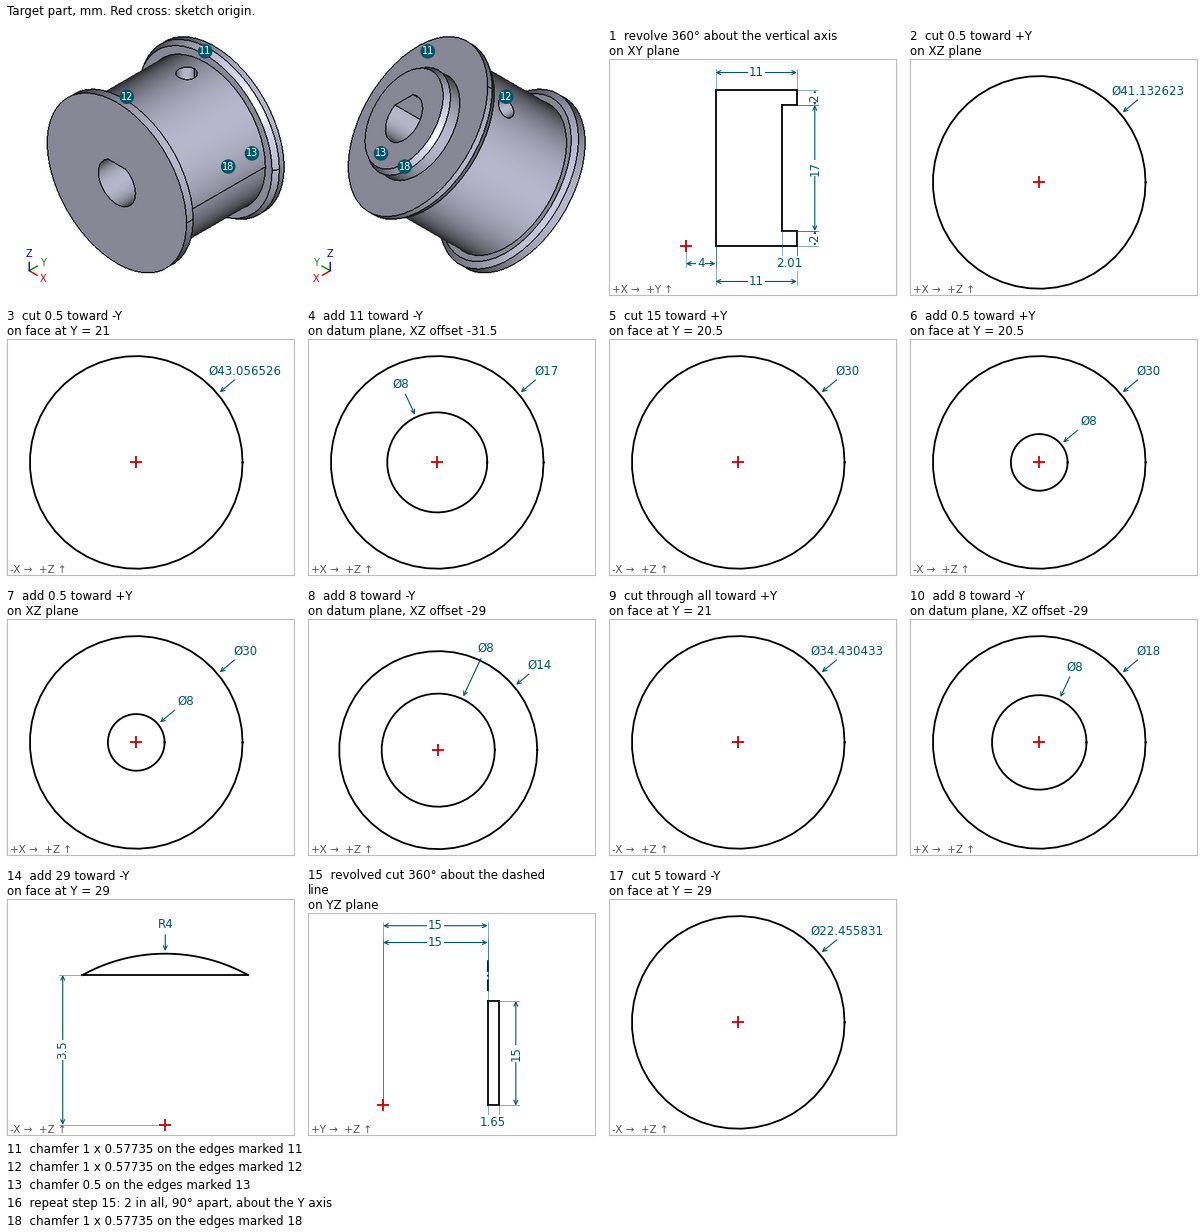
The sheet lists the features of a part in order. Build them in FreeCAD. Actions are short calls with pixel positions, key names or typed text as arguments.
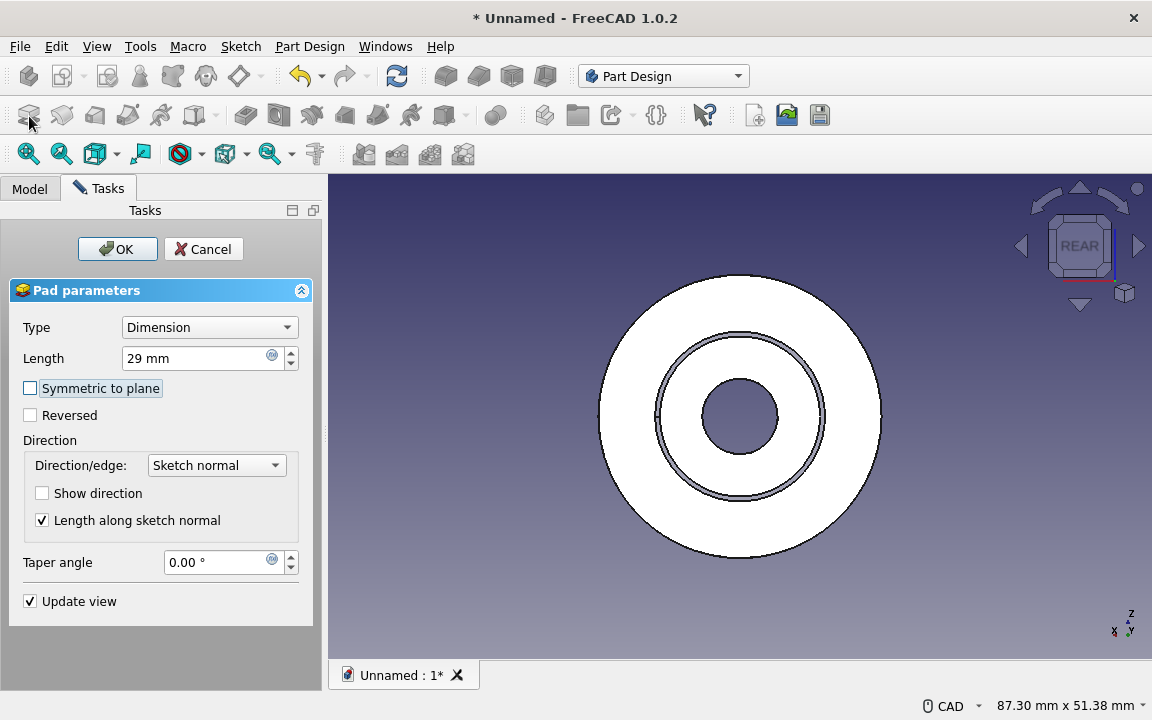
click(31, 415)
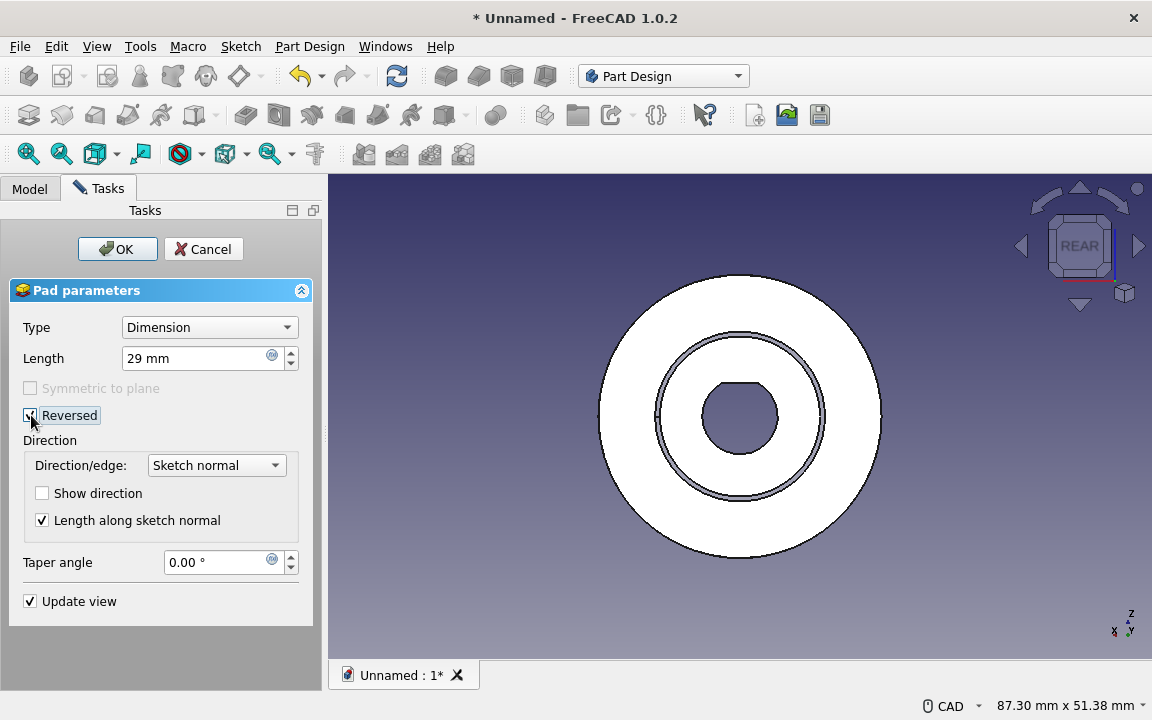
click(118, 249)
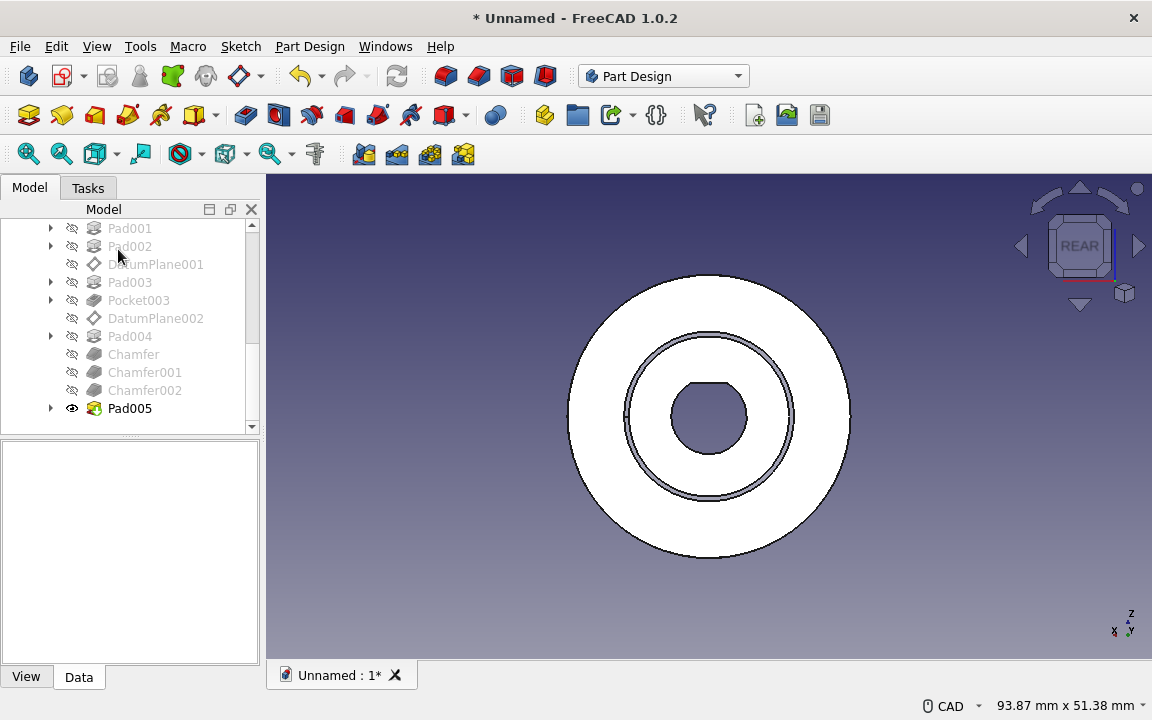
click(62, 76)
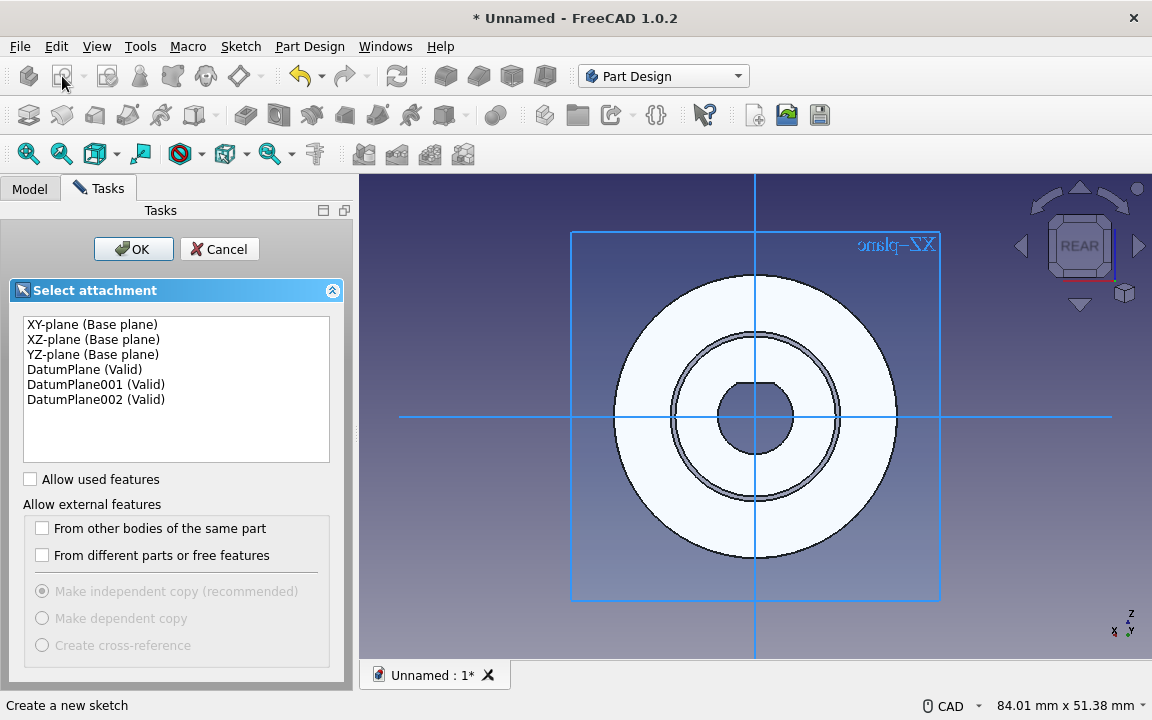
click(84, 354)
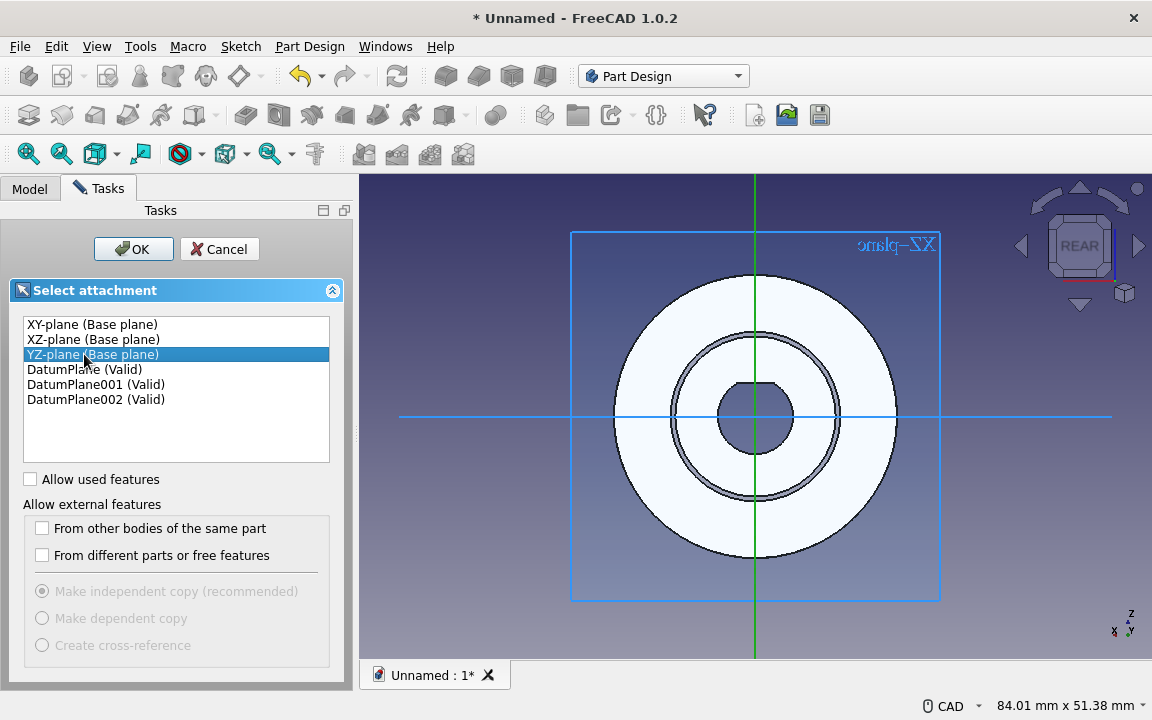
click(134, 249)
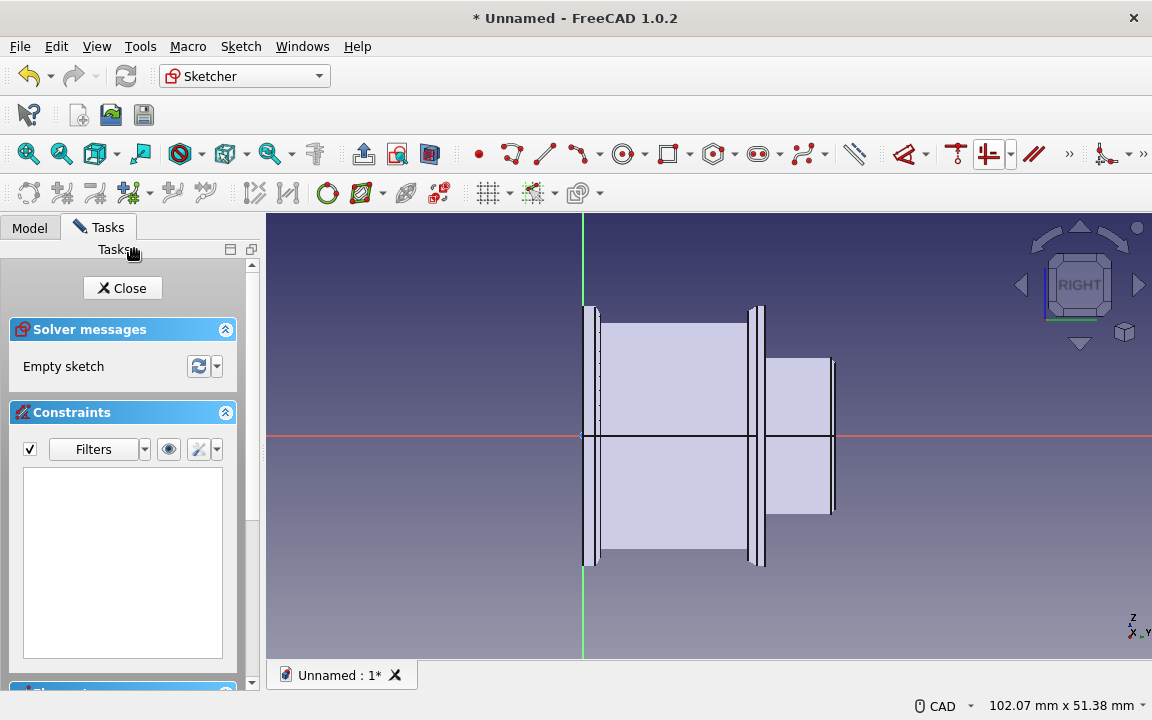
click(430, 154)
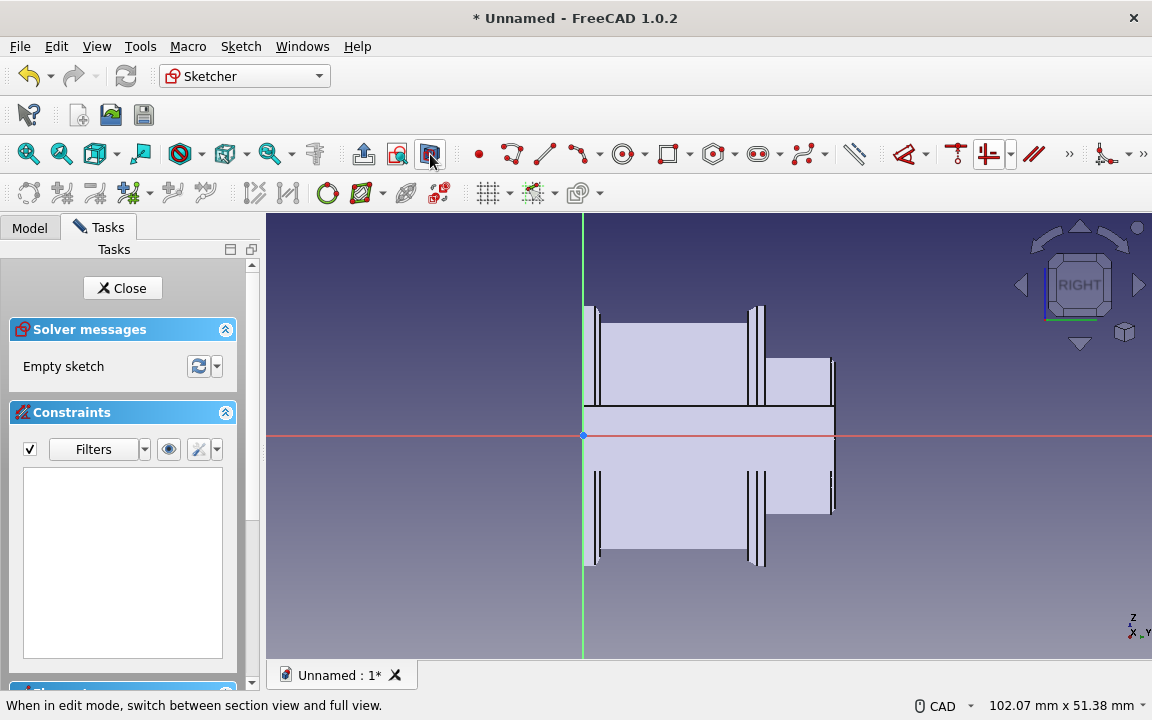
scroll(573, 631, down, 1)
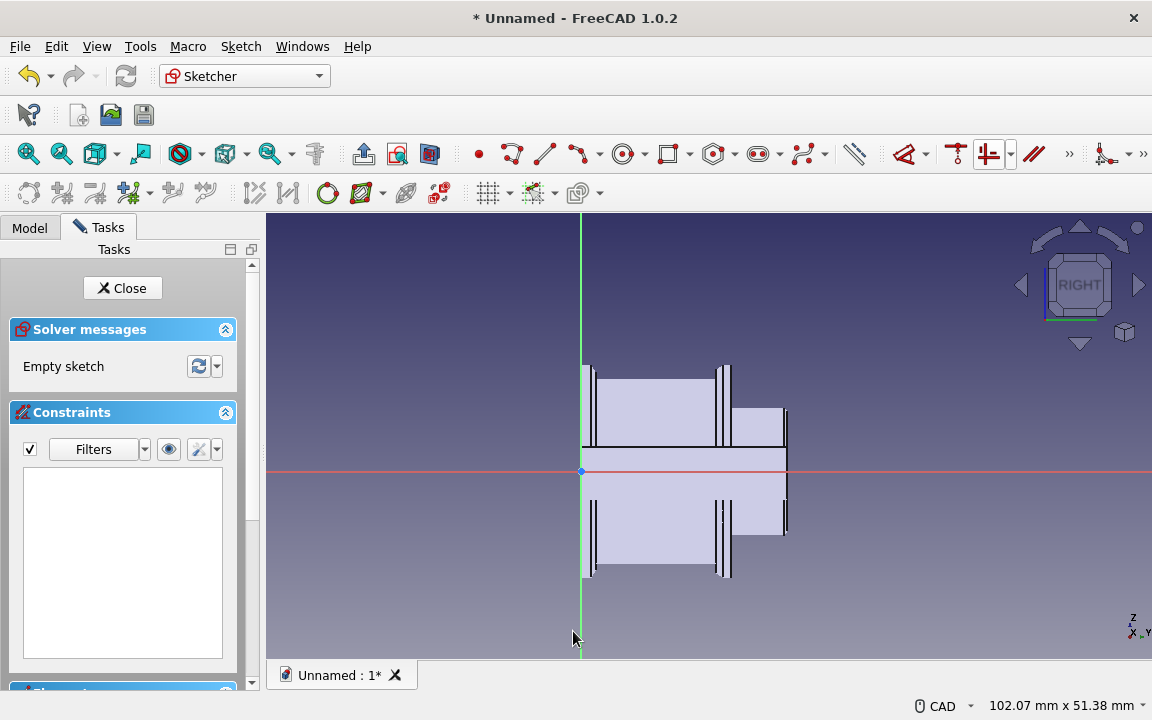
scroll(641, 349, up, 3)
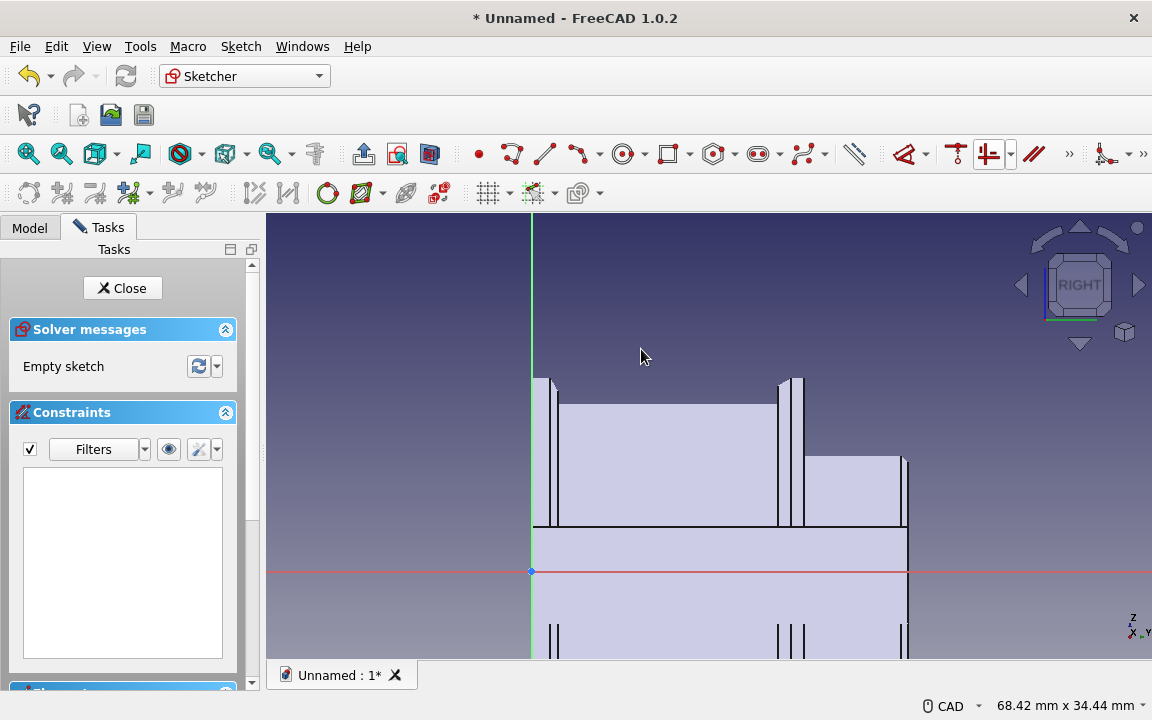
click(668, 154)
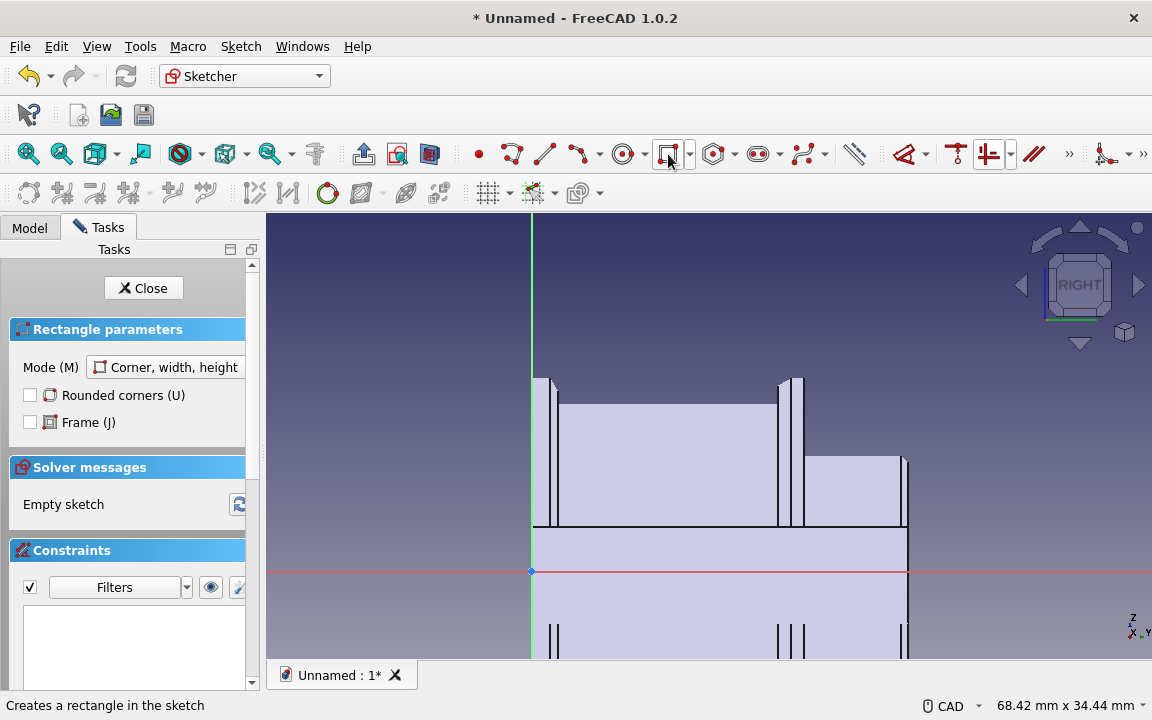
click(726, 378)
click(748, 572)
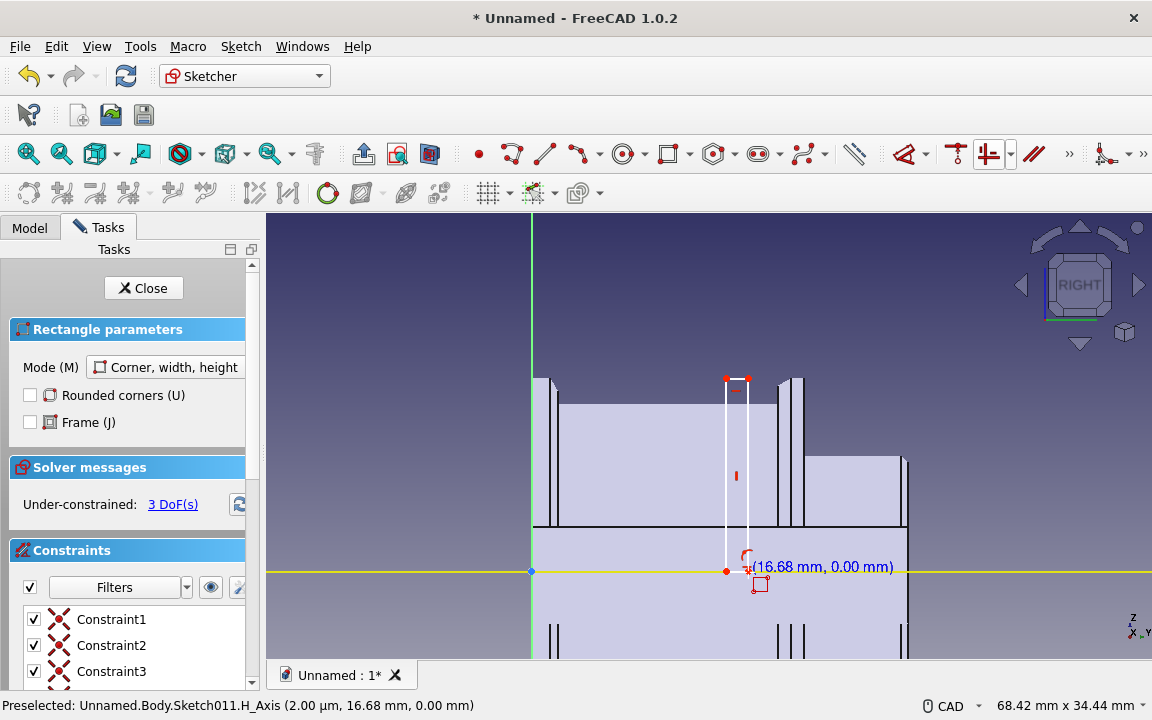
click(545, 154)